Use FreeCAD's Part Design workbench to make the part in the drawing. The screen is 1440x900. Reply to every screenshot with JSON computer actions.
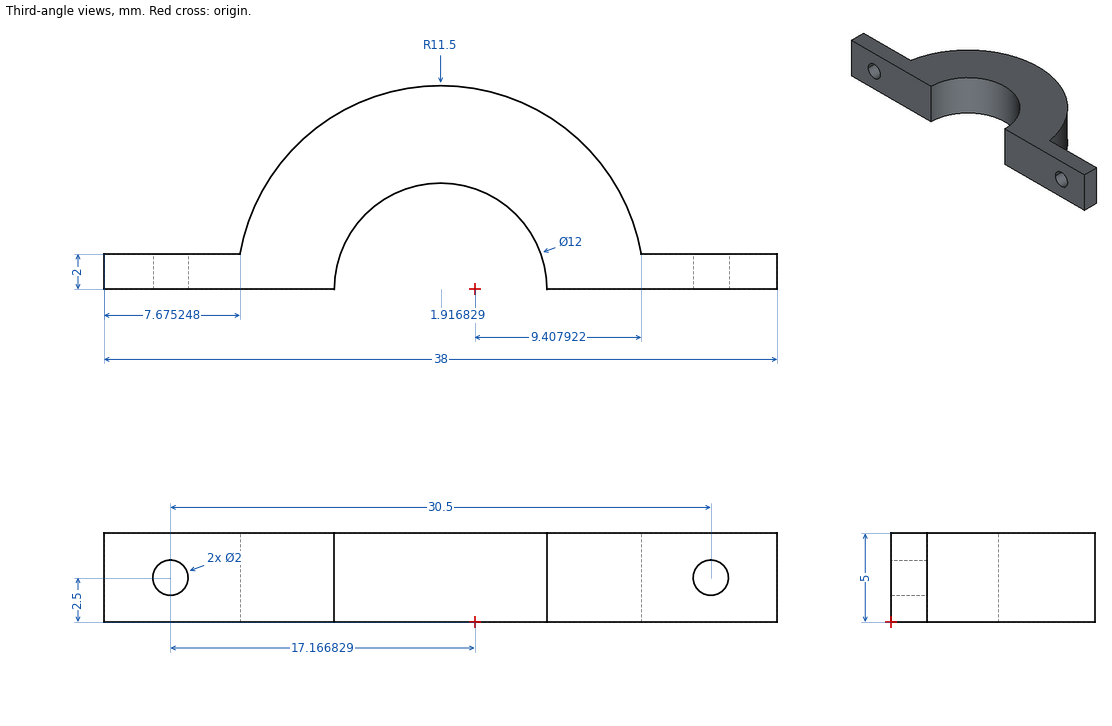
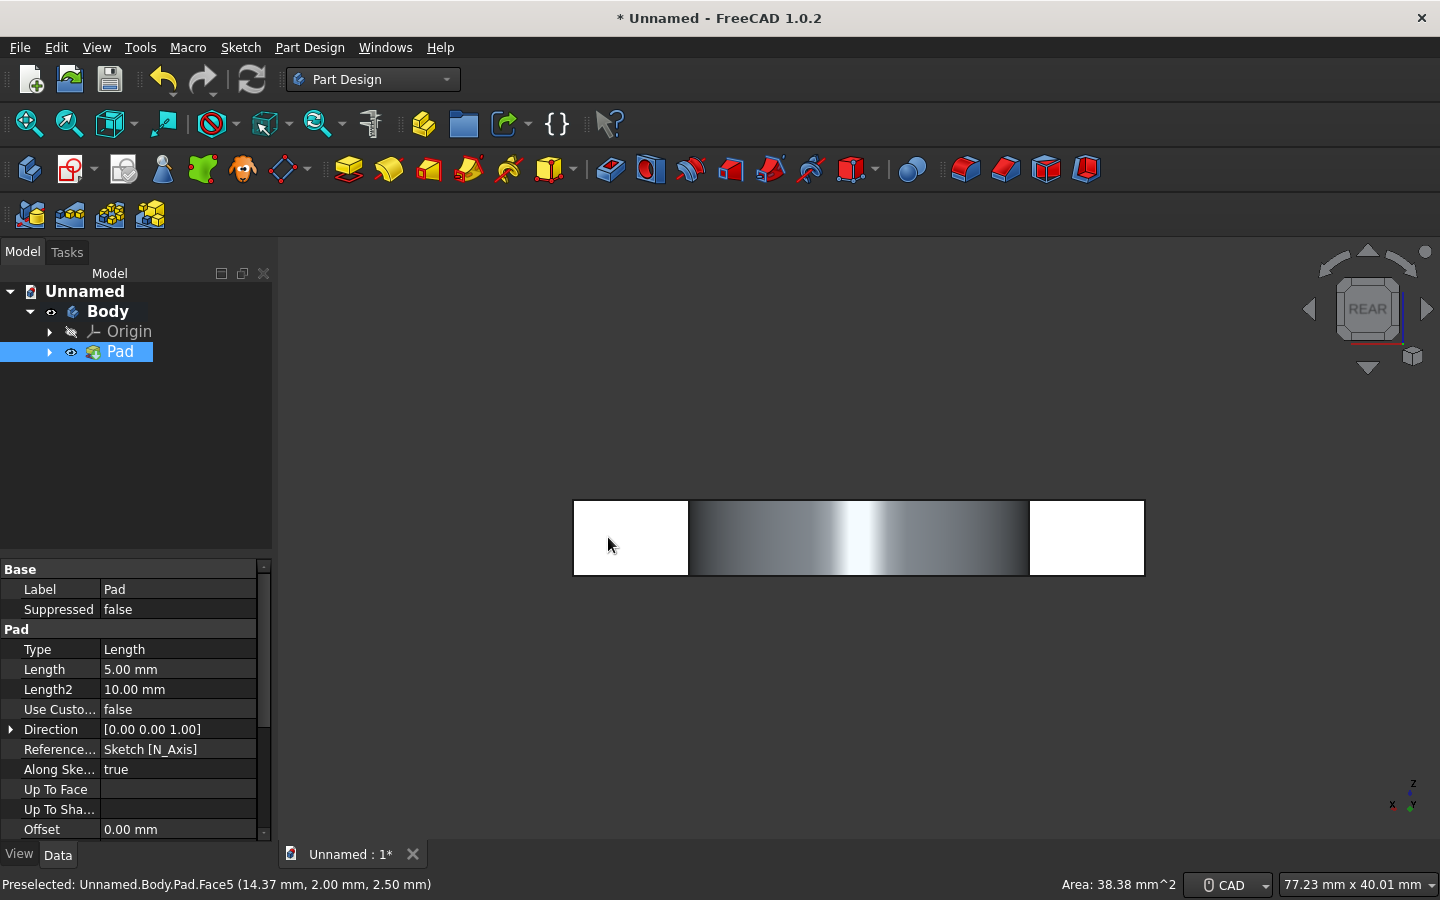
{"action": "left_click", "coordinate": [70, 170]}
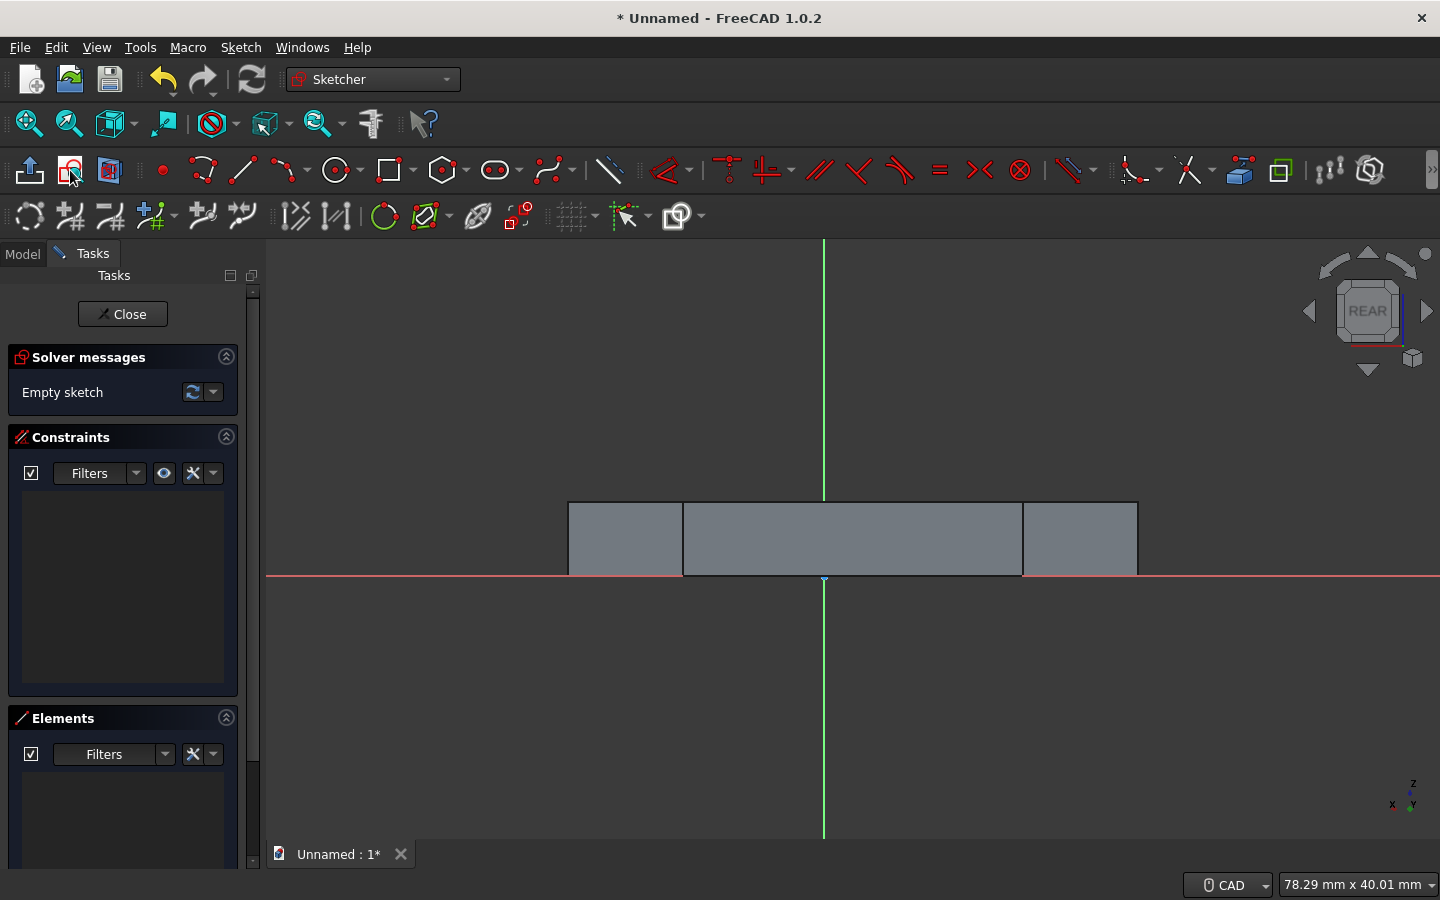
{"action": "scroll", "coordinate": [992, 573], "scroll_direction": "up", "scroll_amount": 2}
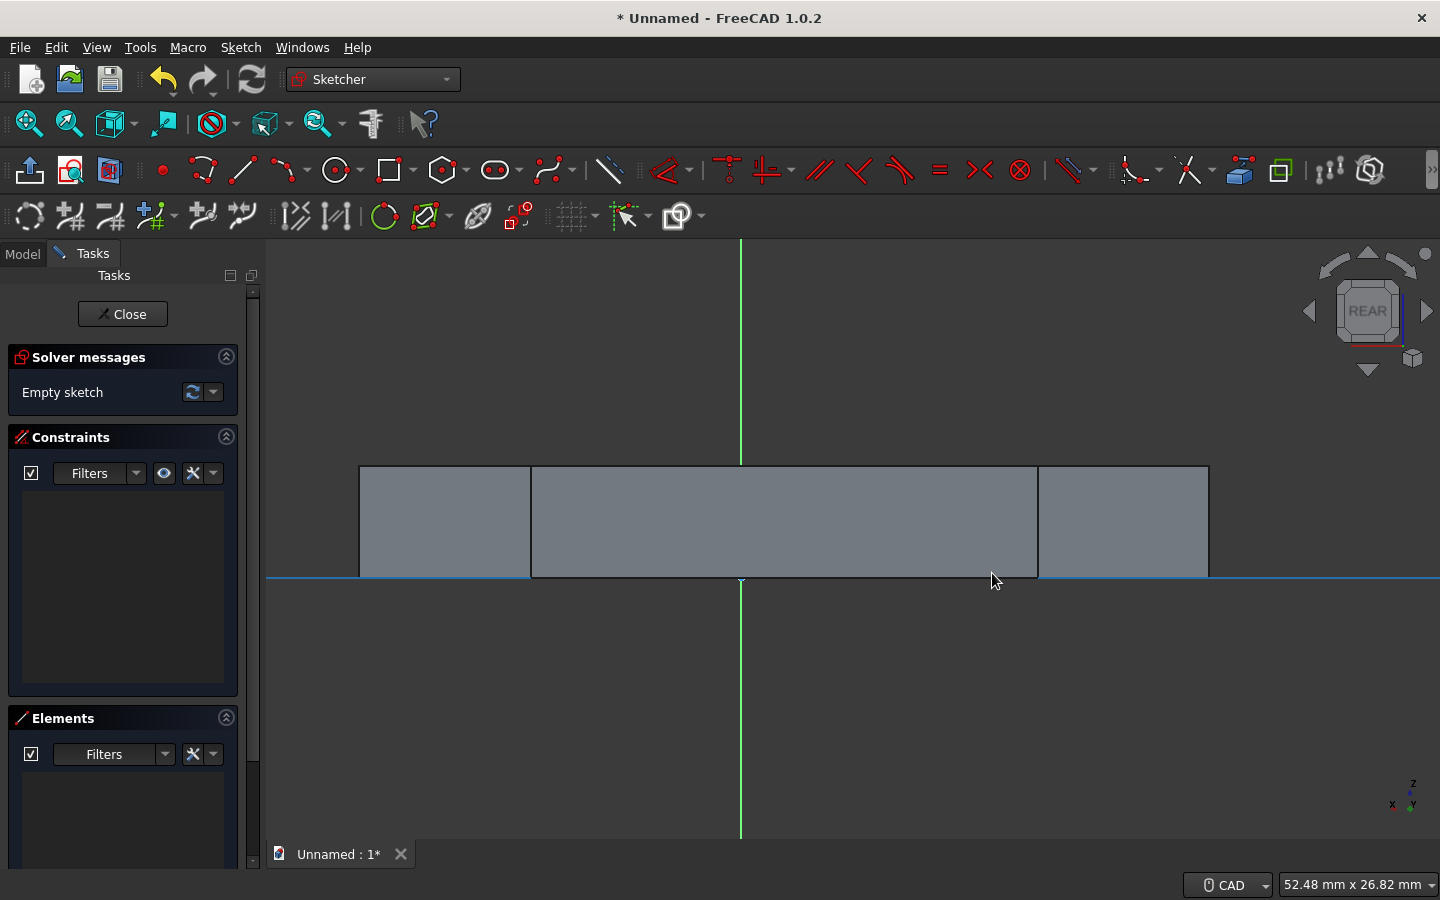
{"action": "left_click", "coordinate": [336, 170]}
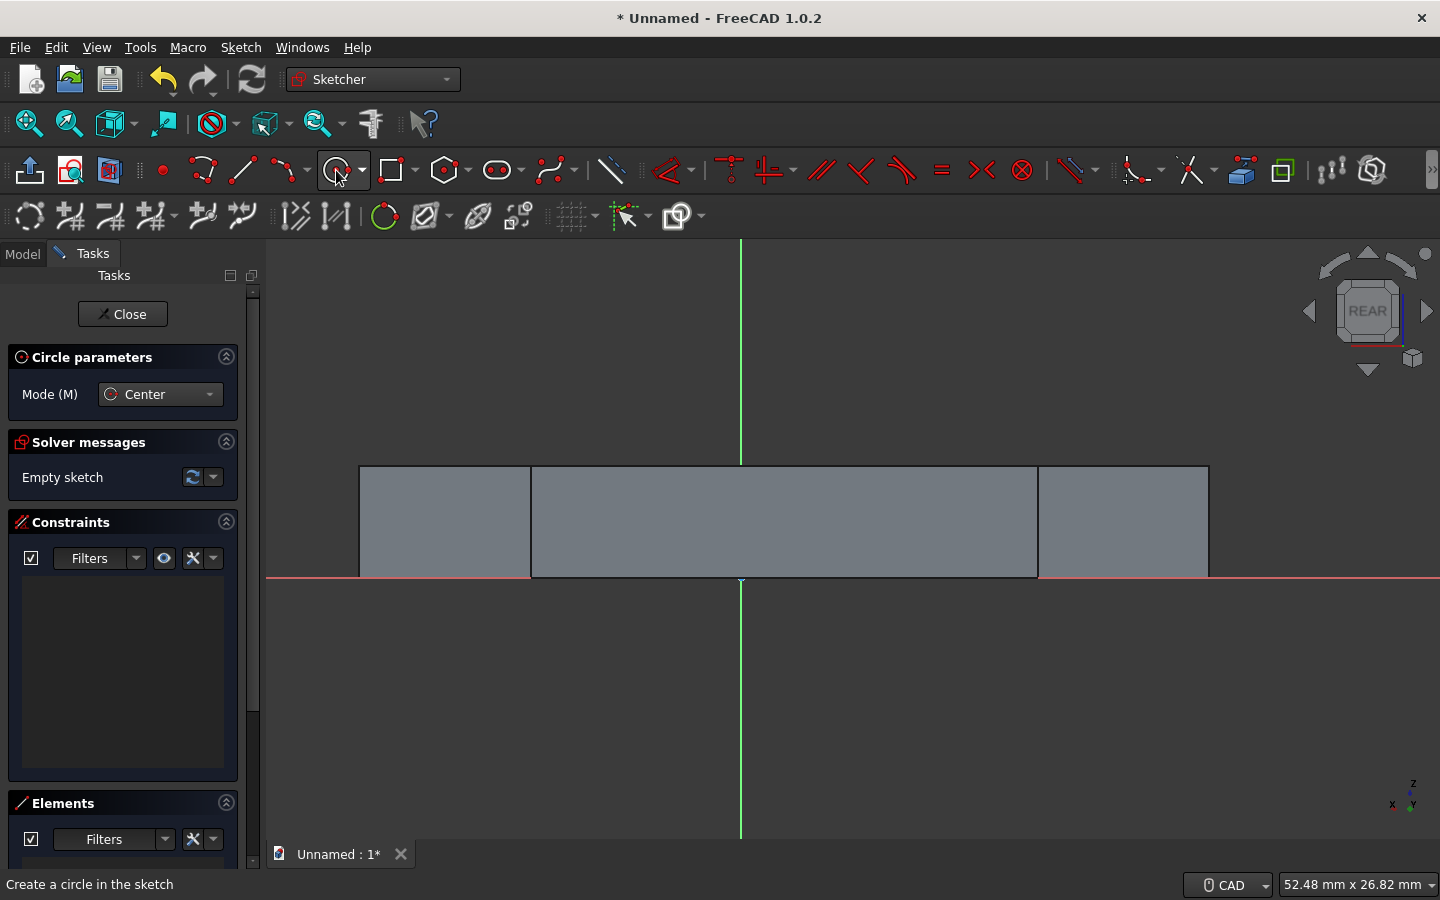
{"action": "left_click", "coordinate": [1125, 522]}
{"action": "left_click", "coordinate": [1141, 506]}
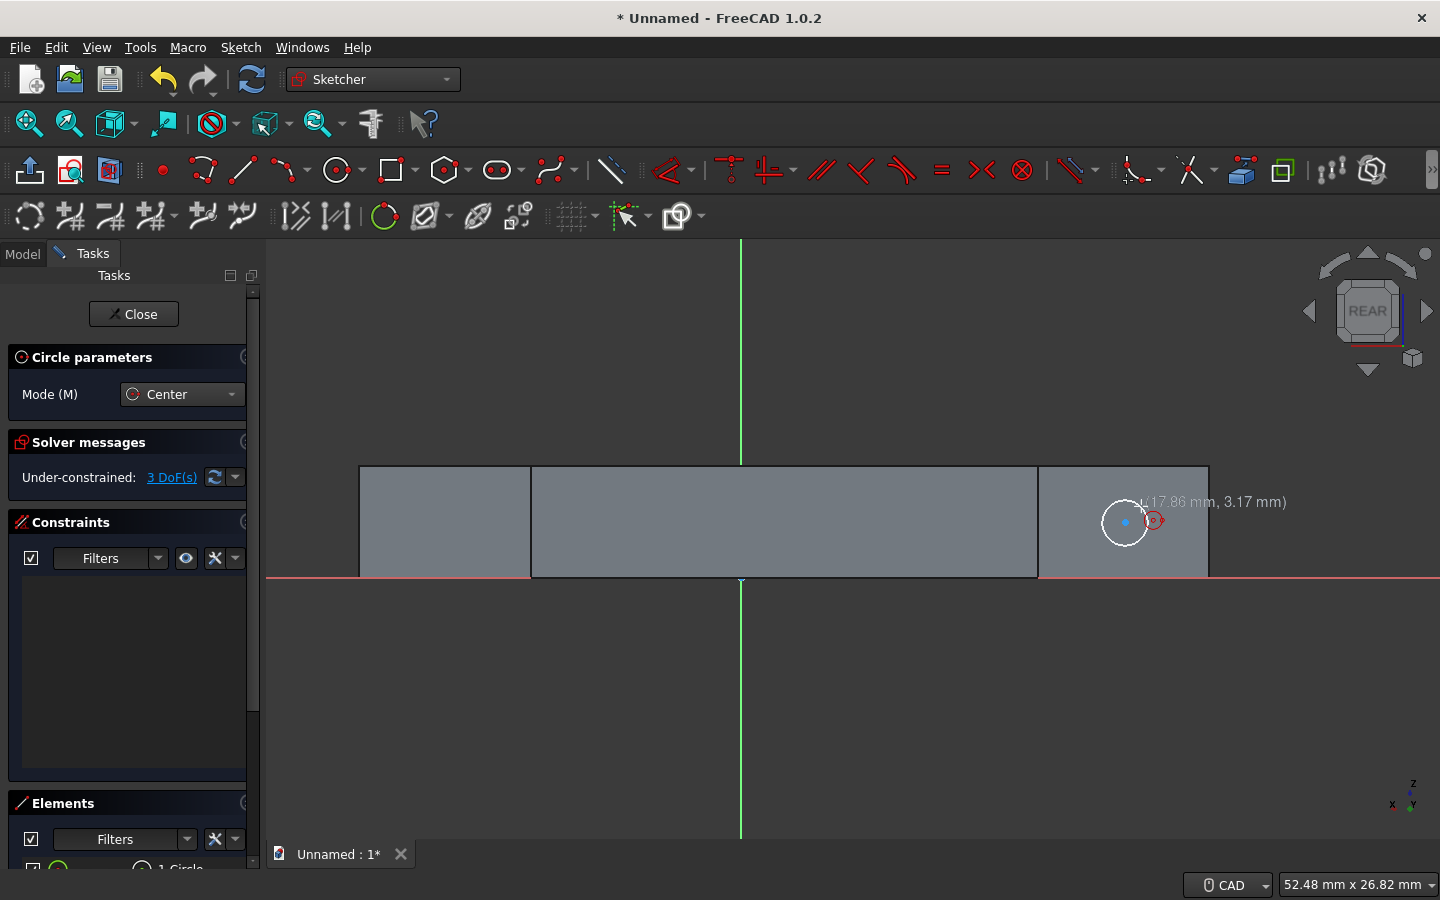
{"action": "left_click", "coordinate": [443, 522]}
{"action": "left_click", "coordinate": [459, 506]}
{"action": "key", "text": "Escape"}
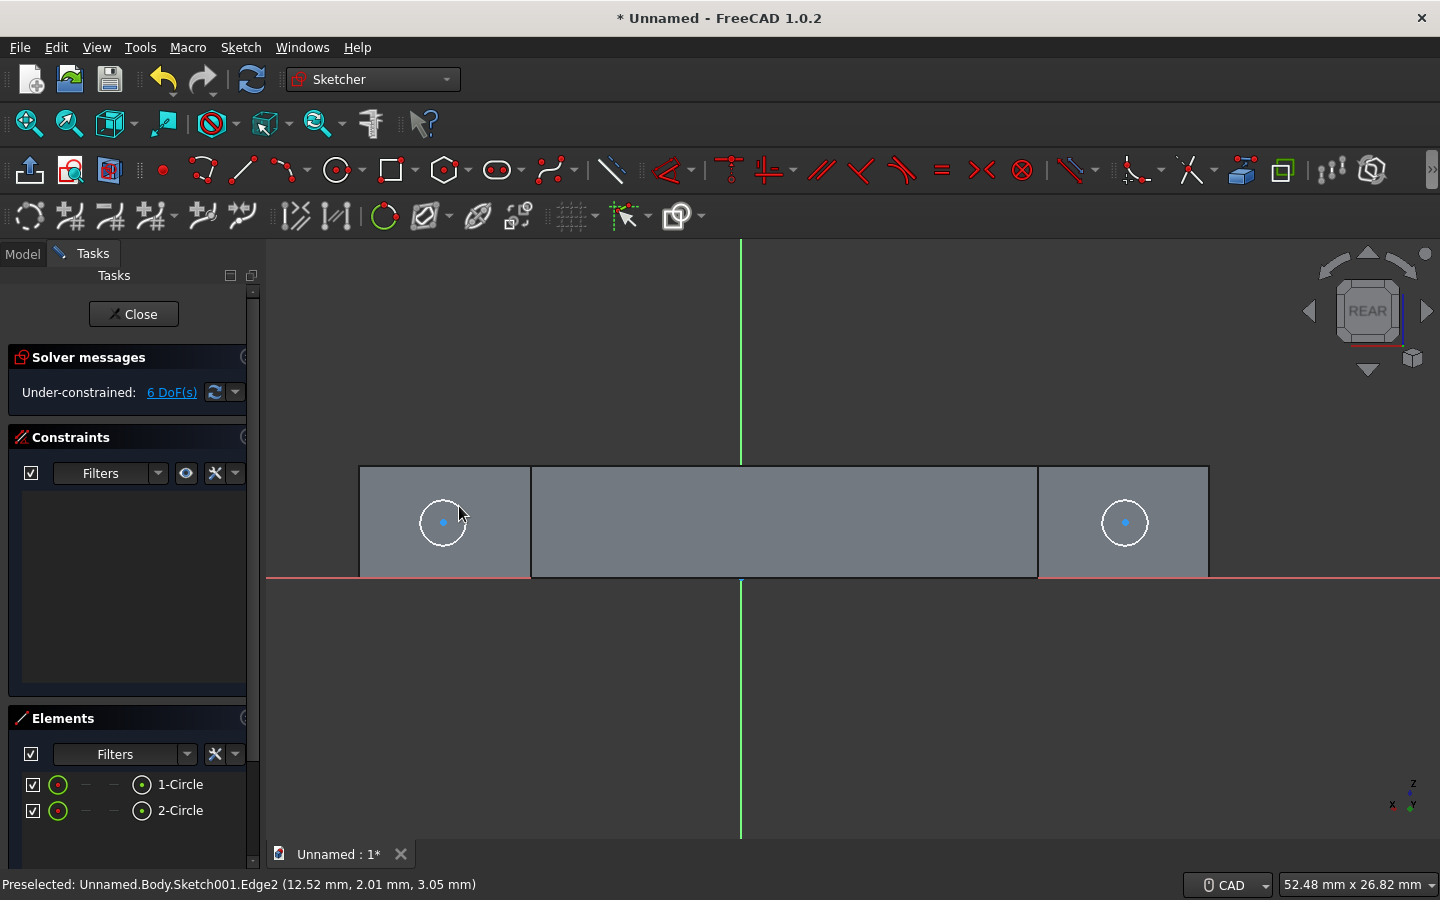
{"action": "left_click", "coordinate": [1141, 507]}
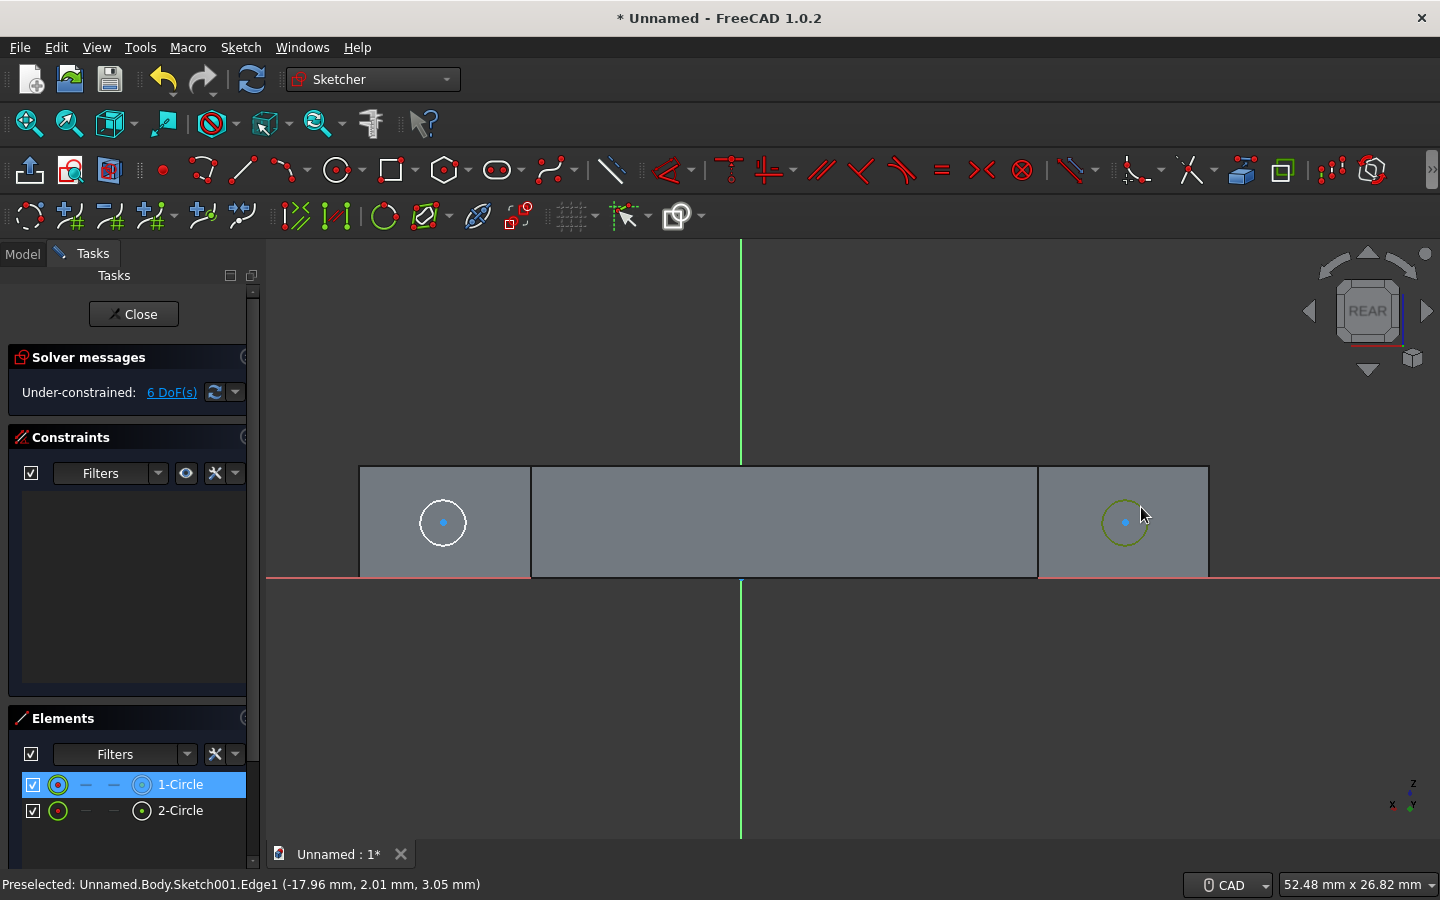
{"action": "left_click", "coordinate": [459, 507]}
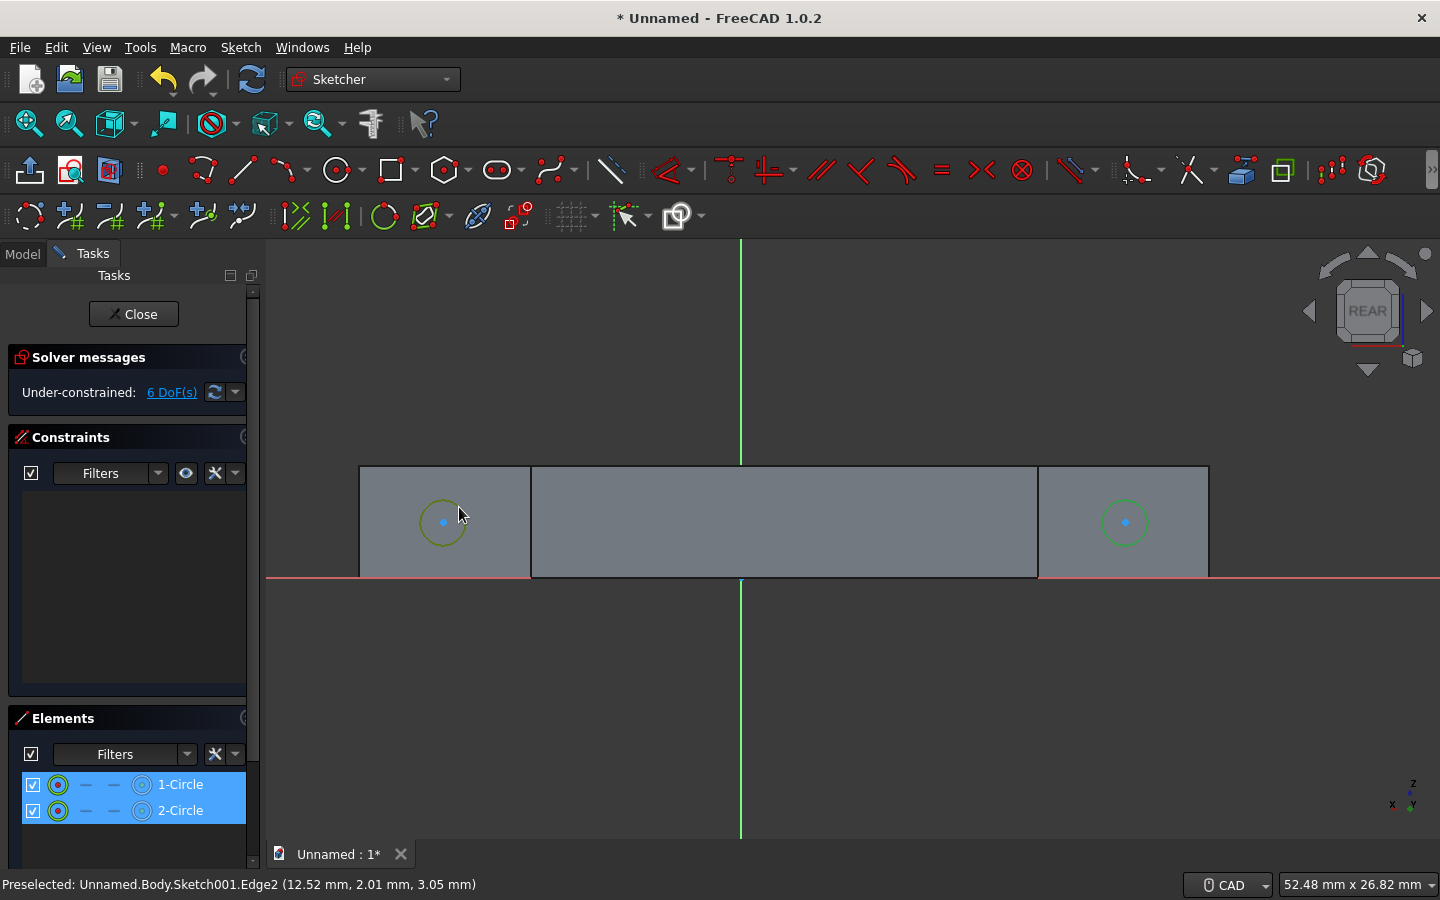
{"action": "key", "text": "e"}